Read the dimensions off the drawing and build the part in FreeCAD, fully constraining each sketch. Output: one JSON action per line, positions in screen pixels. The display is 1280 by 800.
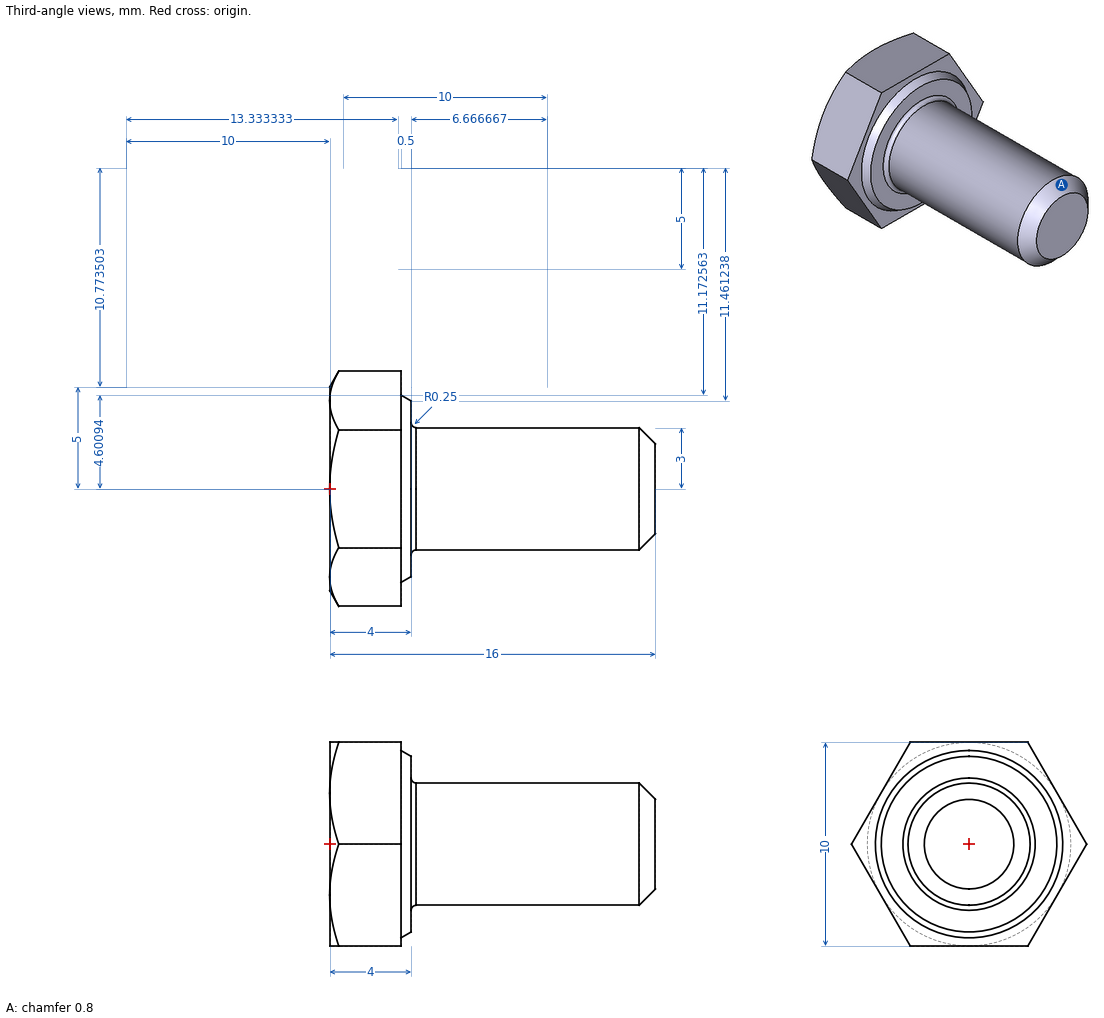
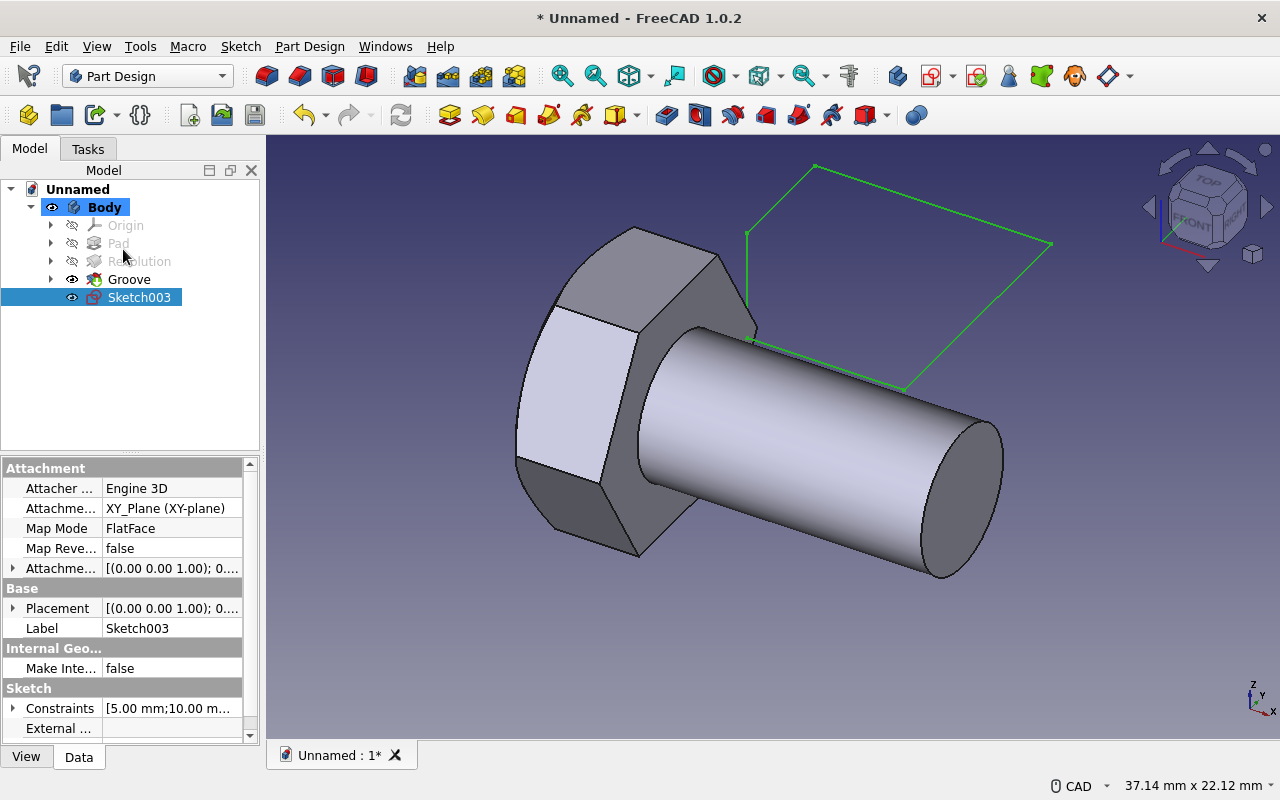
{"action": "left_click", "coordinate": [733, 116]}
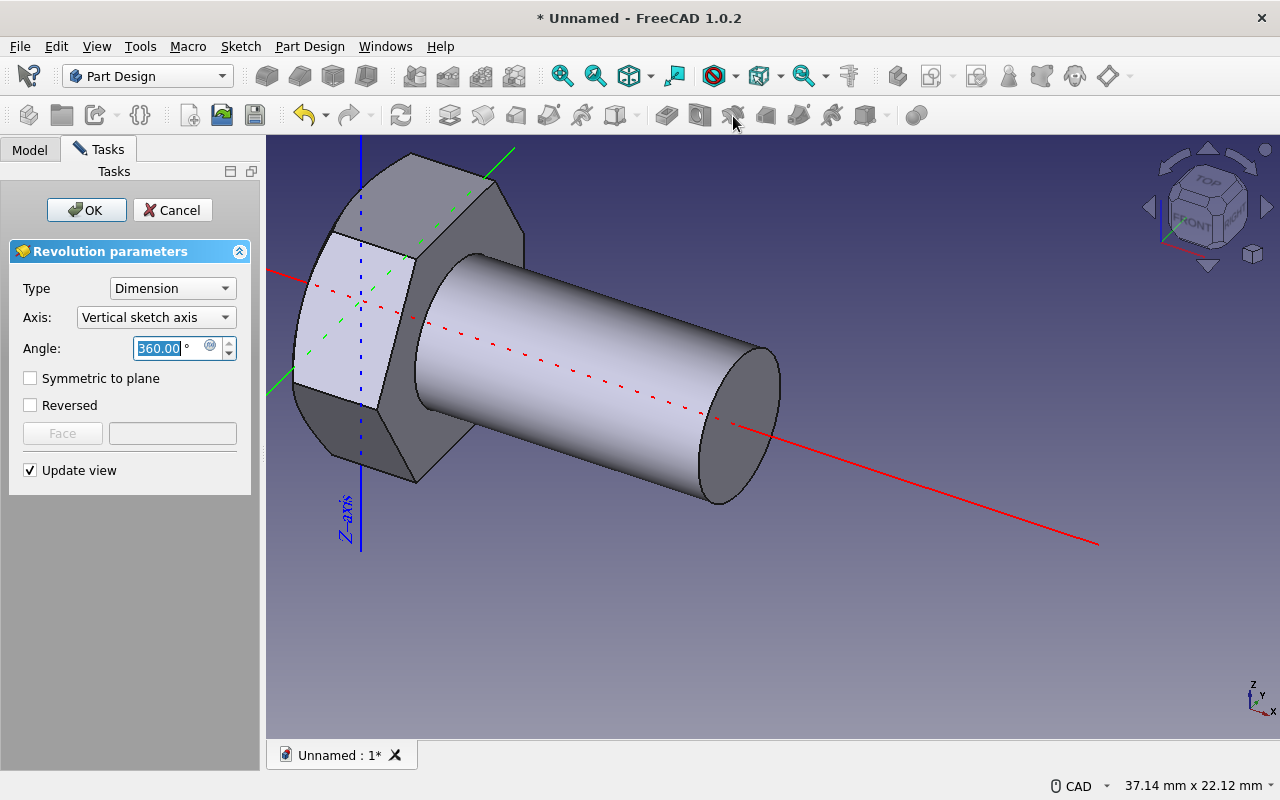
{"action": "left_click", "coordinate": [157, 318]}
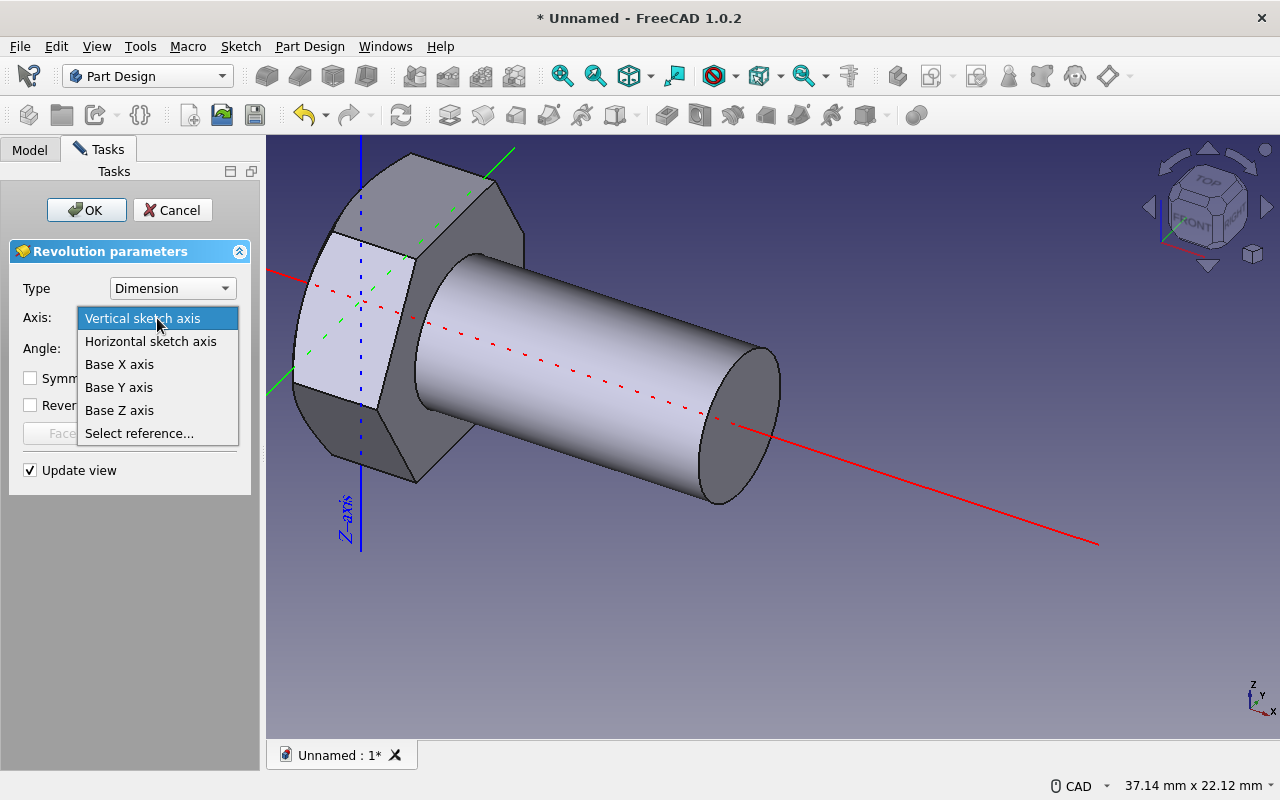
{"action": "left_click", "coordinate": [156, 342]}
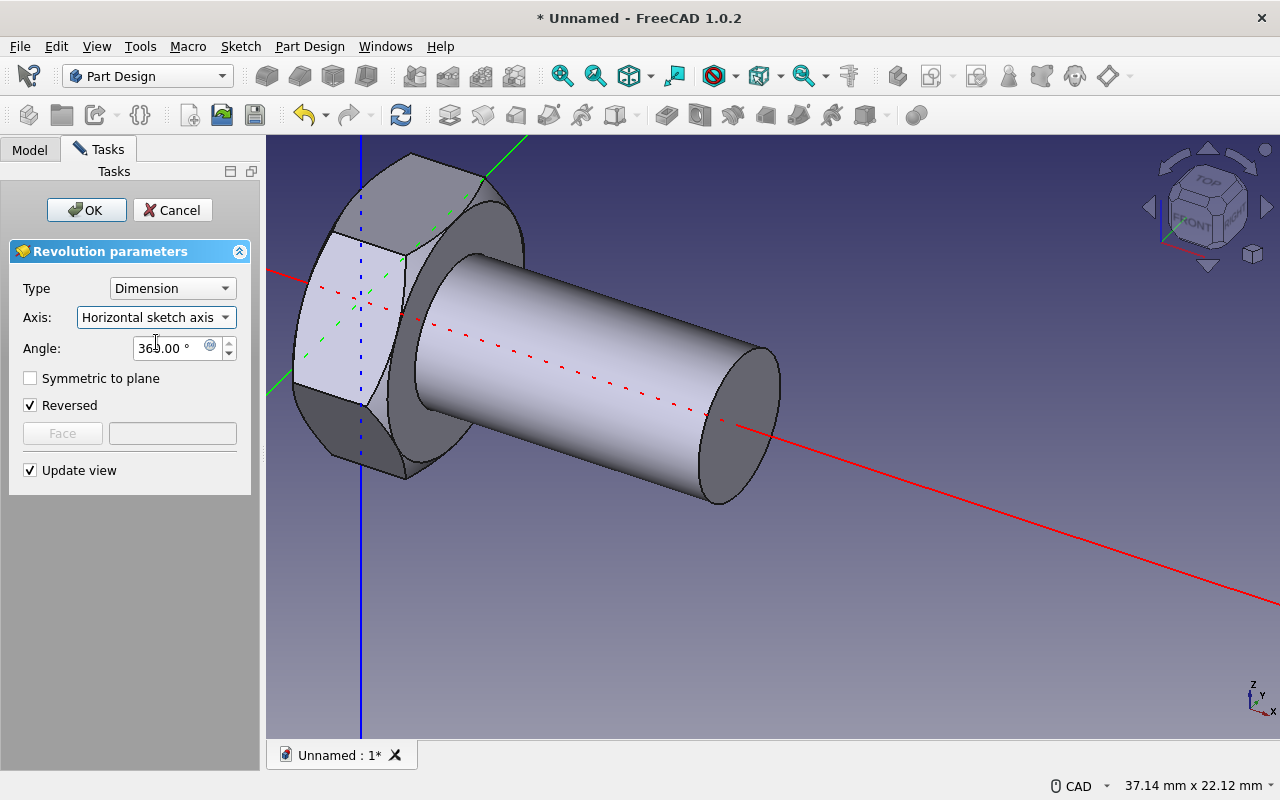
{"action": "left_click", "coordinate": [87, 210]}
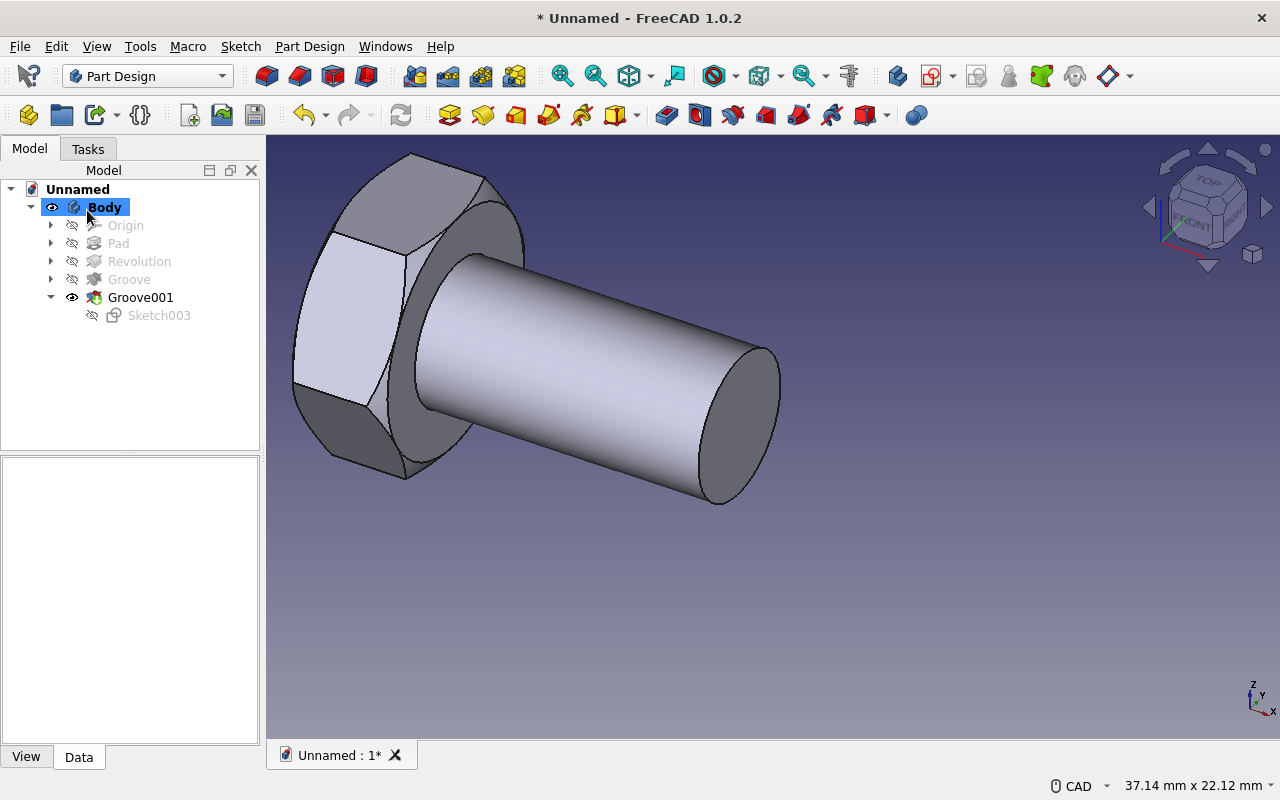
{"action": "left_click", "coordinate": [563, 76]}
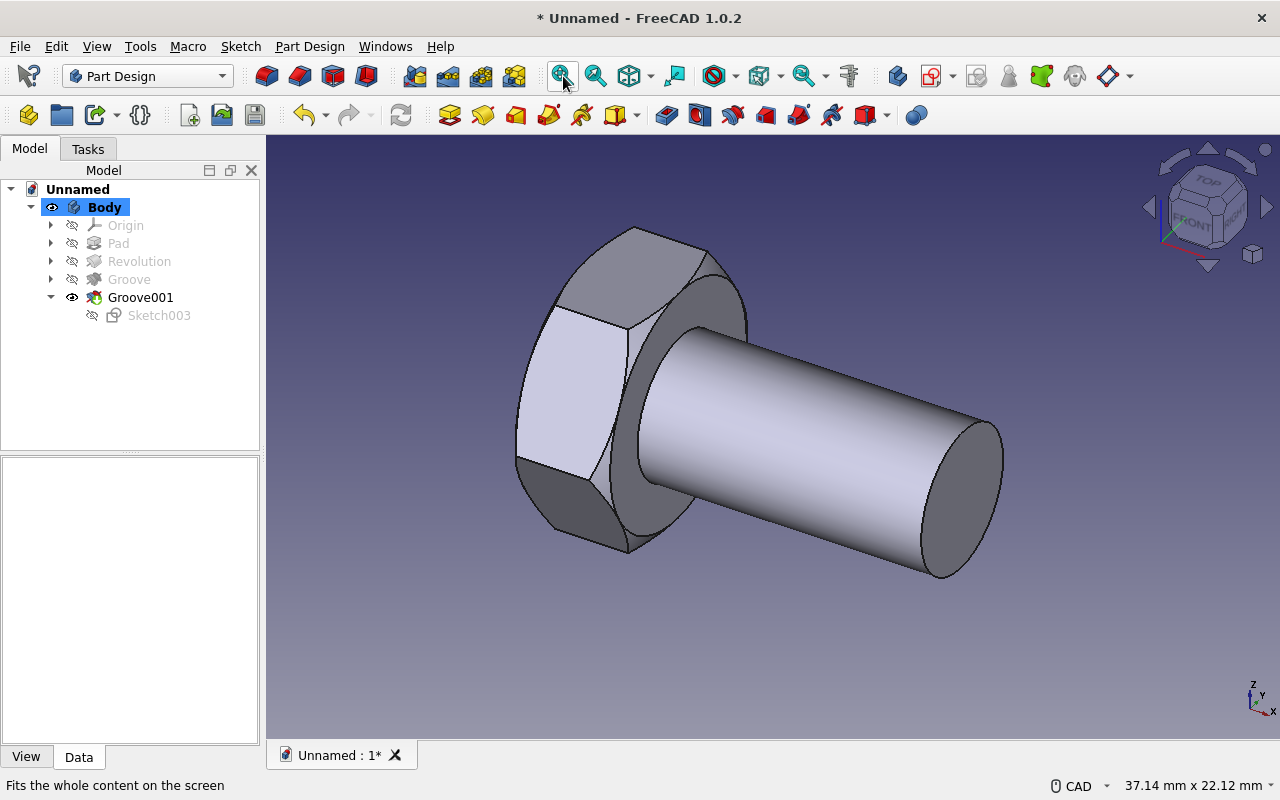
{"action": "left_click", "coordinate": [930, 76]}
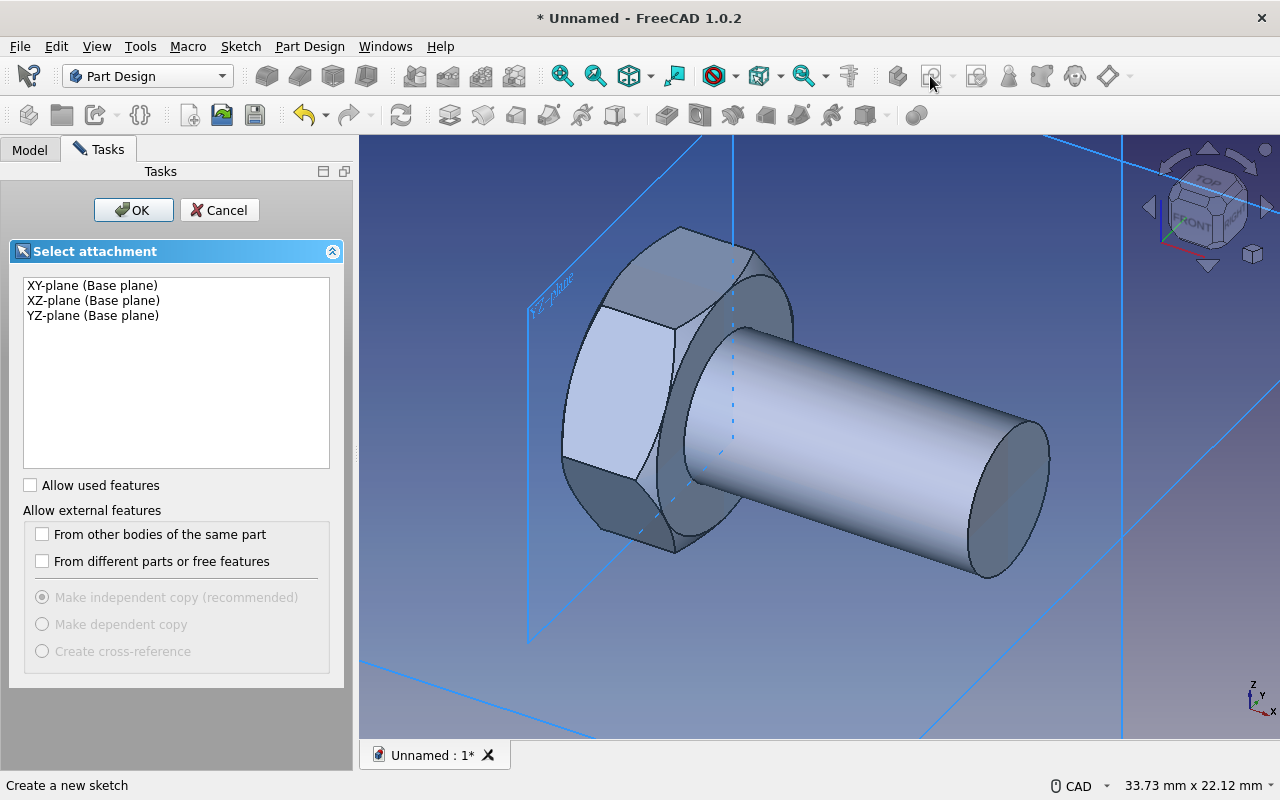
{"action": "left_click", "coordinate": [84, 286]}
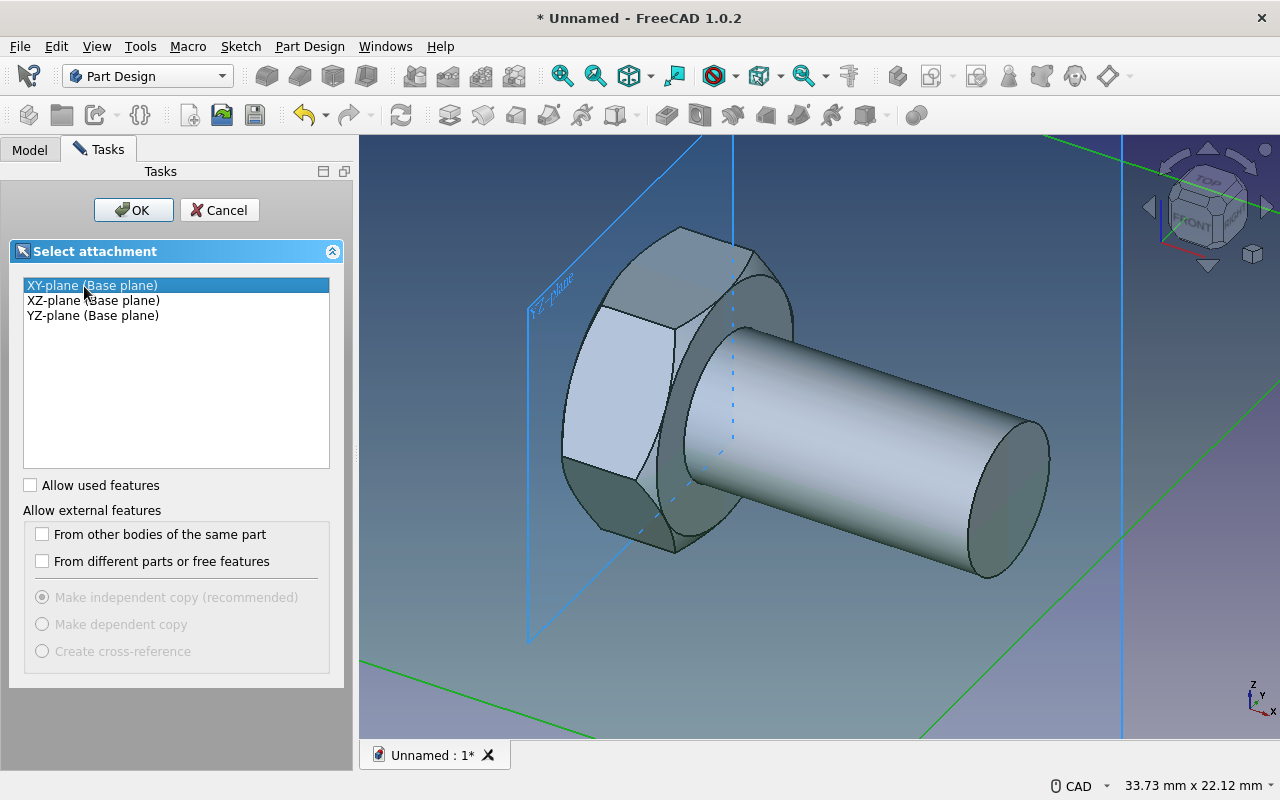
{"action": "left_click", "coordinate": [134, 210]}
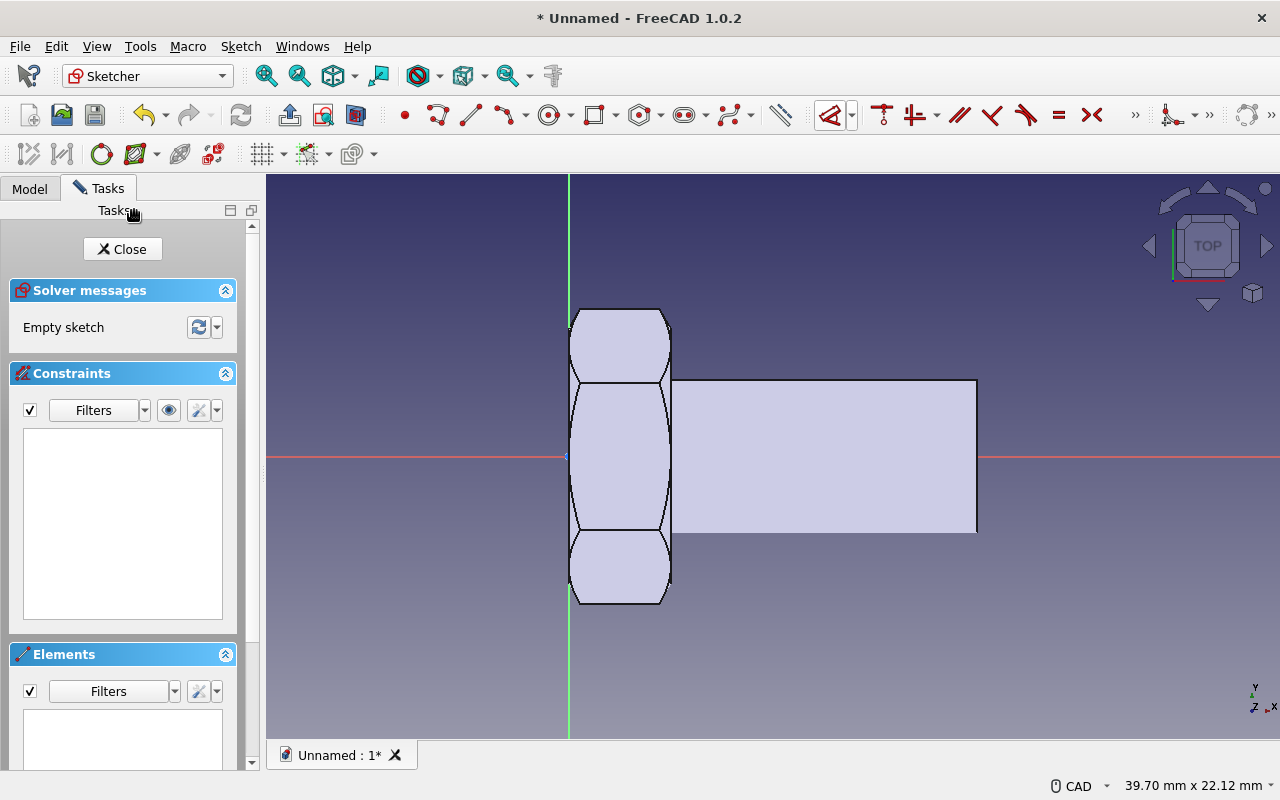
{"action": "left_click", "coordinate": [356, 116]}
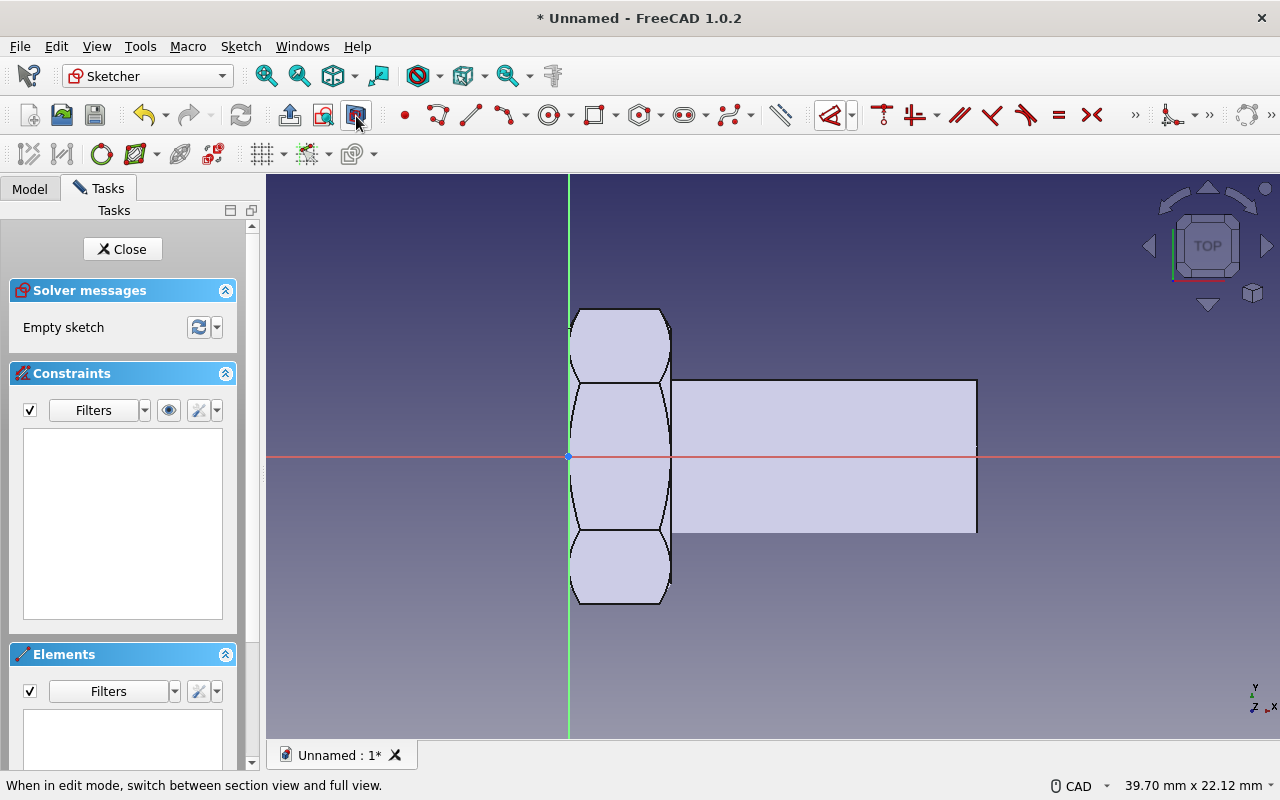
{"action": "scroll", "coordinate": [877, 711], "scroll_direction": "down", "scroll_amount": 2}